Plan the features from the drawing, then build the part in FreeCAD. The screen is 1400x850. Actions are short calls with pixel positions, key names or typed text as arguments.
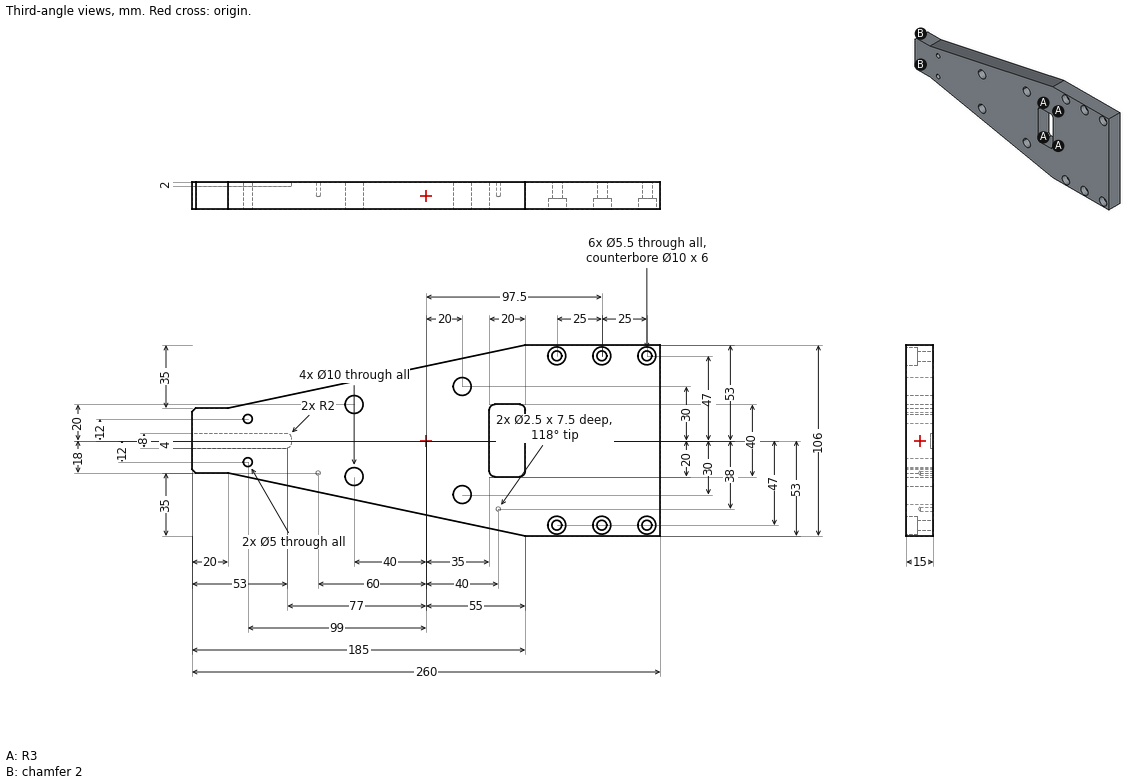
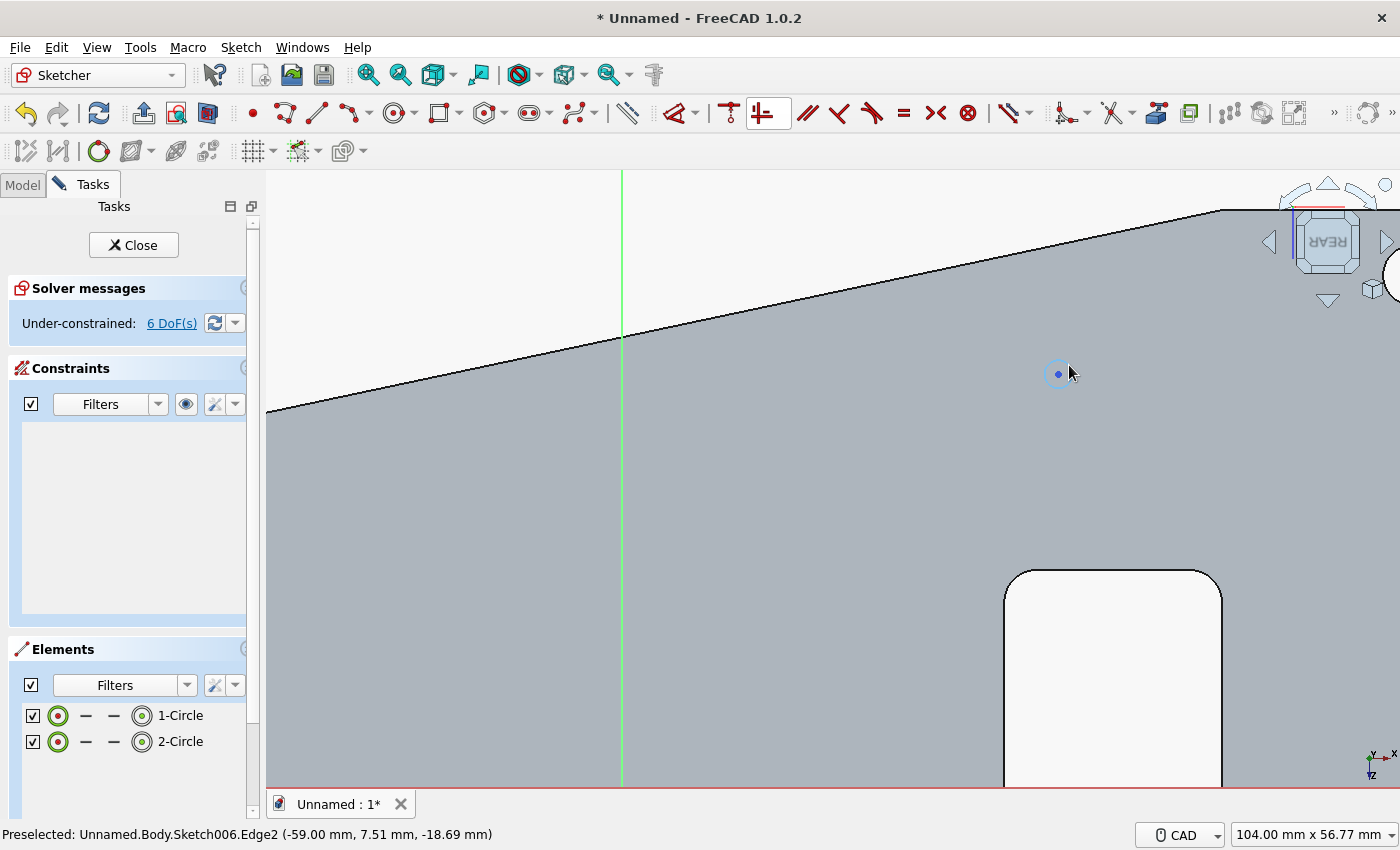
click(1068, 364)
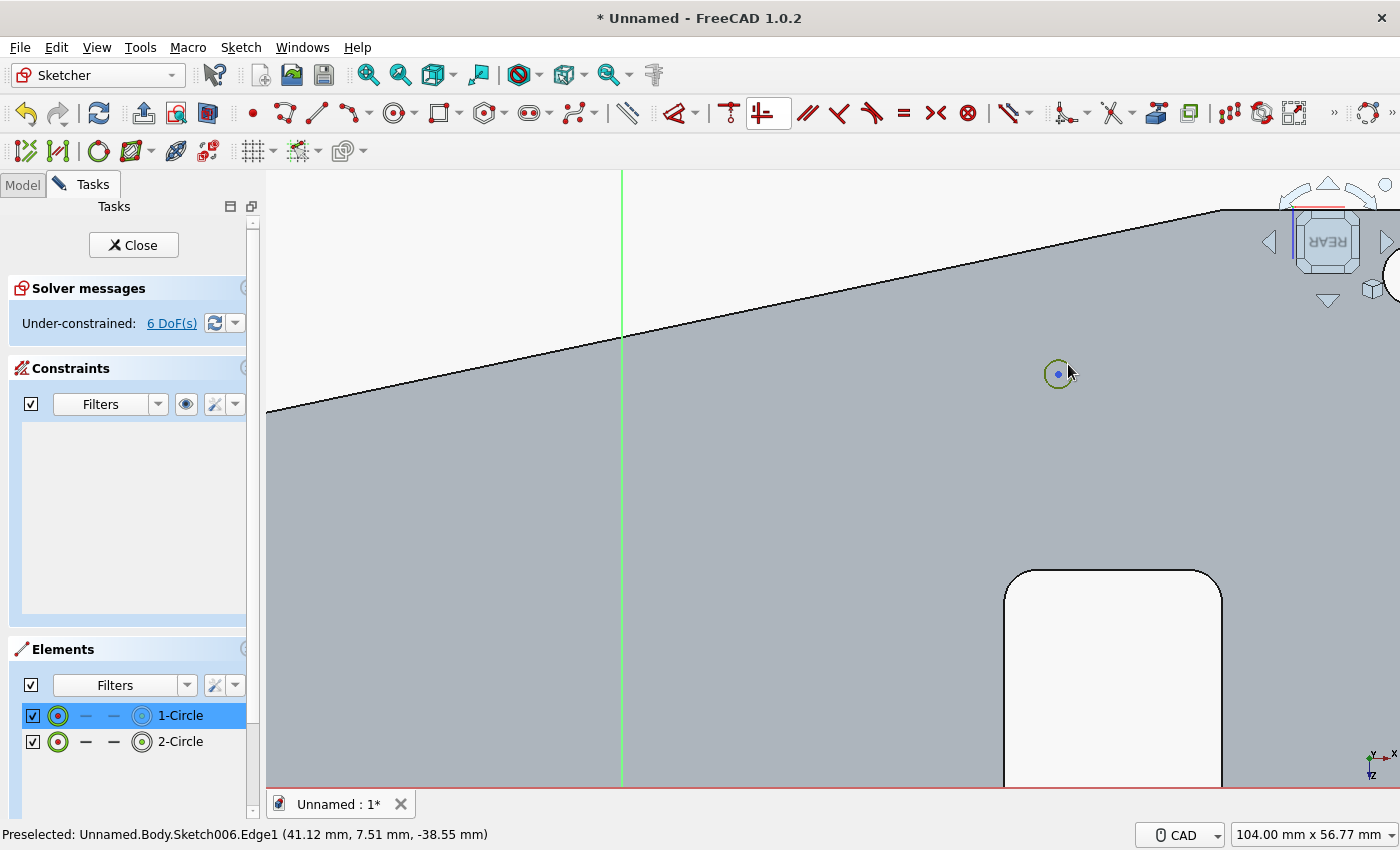
scroll(1070, 365, down, 3)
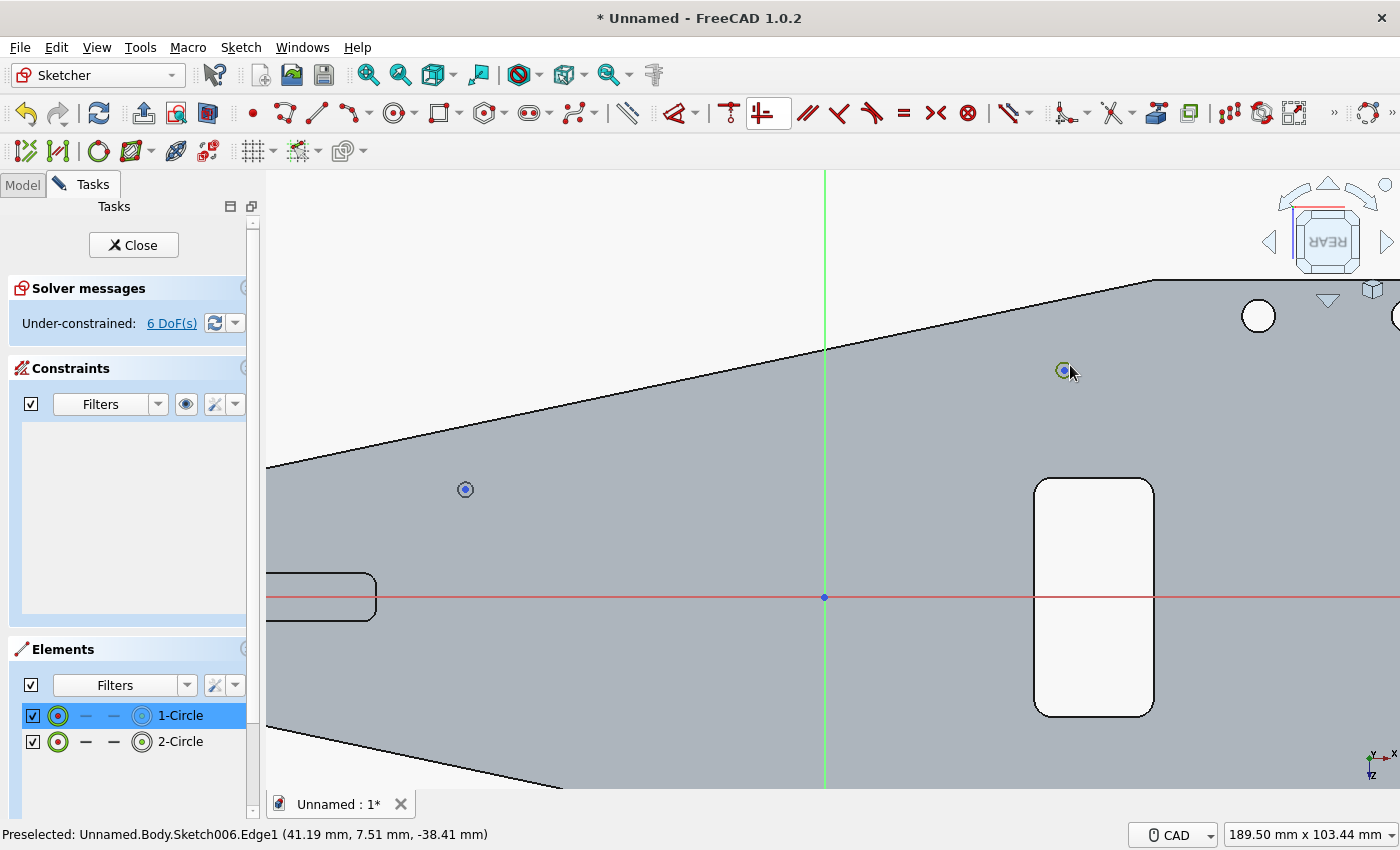
scroll(471, 484, up, 4)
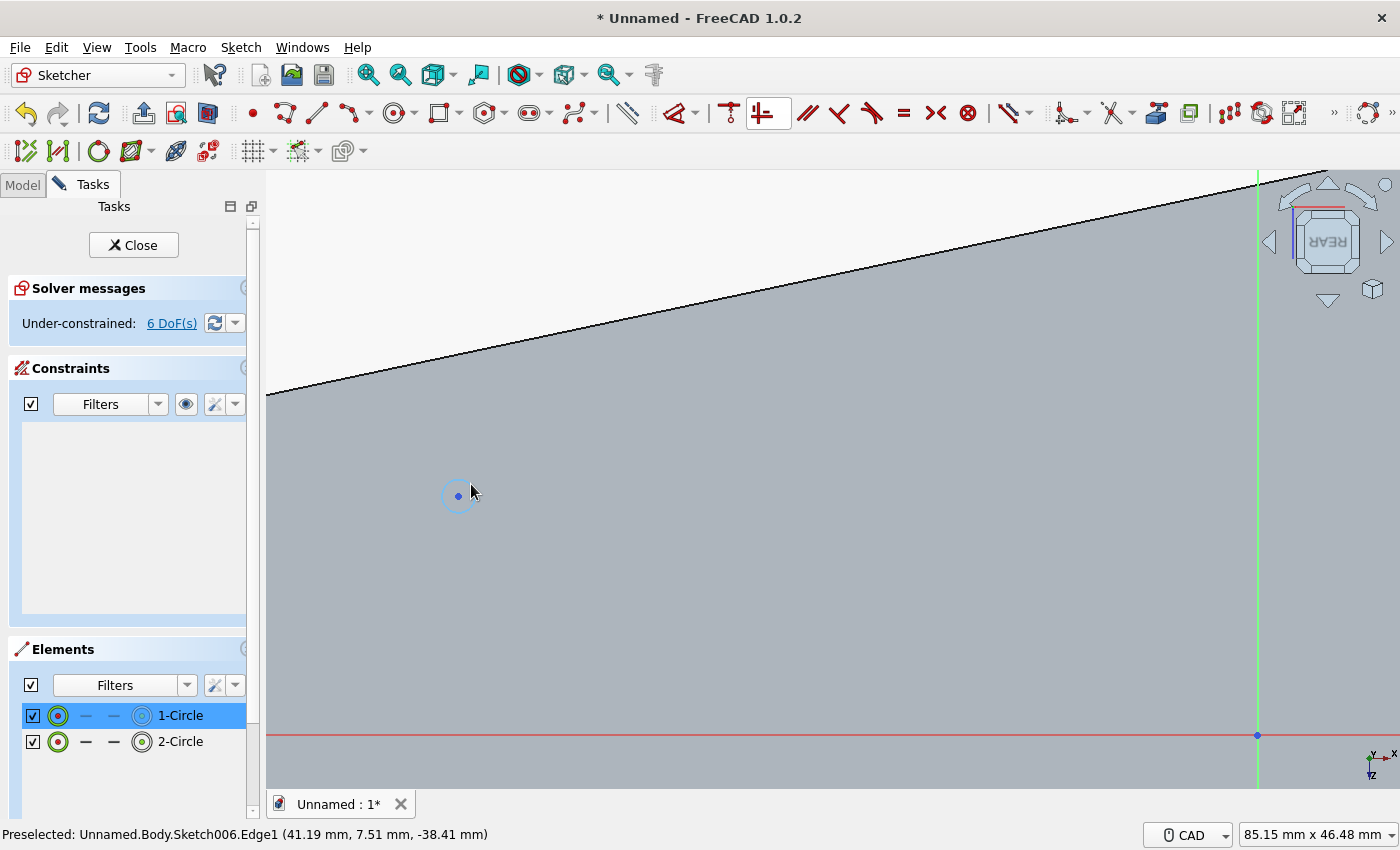
click(470, 484)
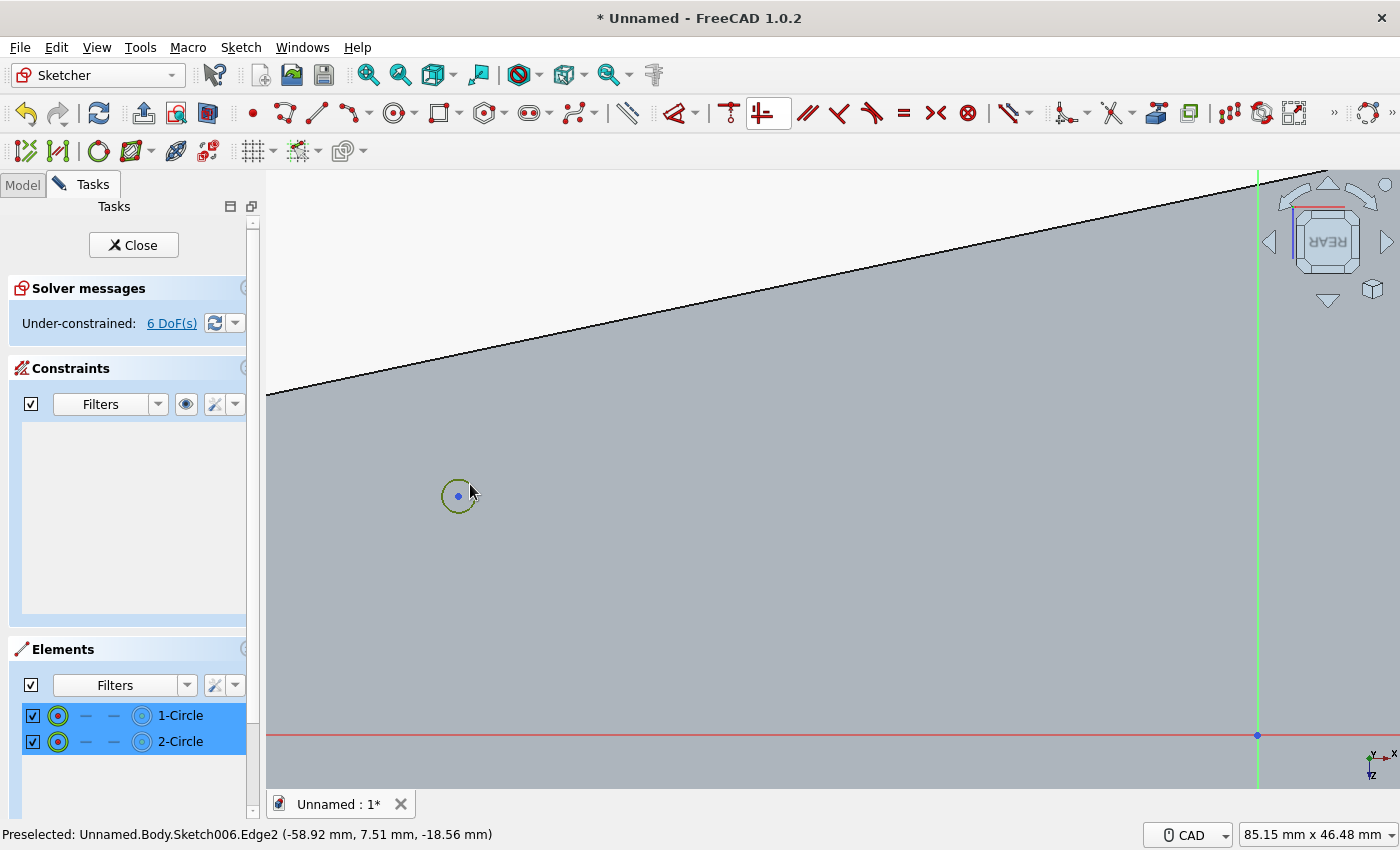
click(904, 114)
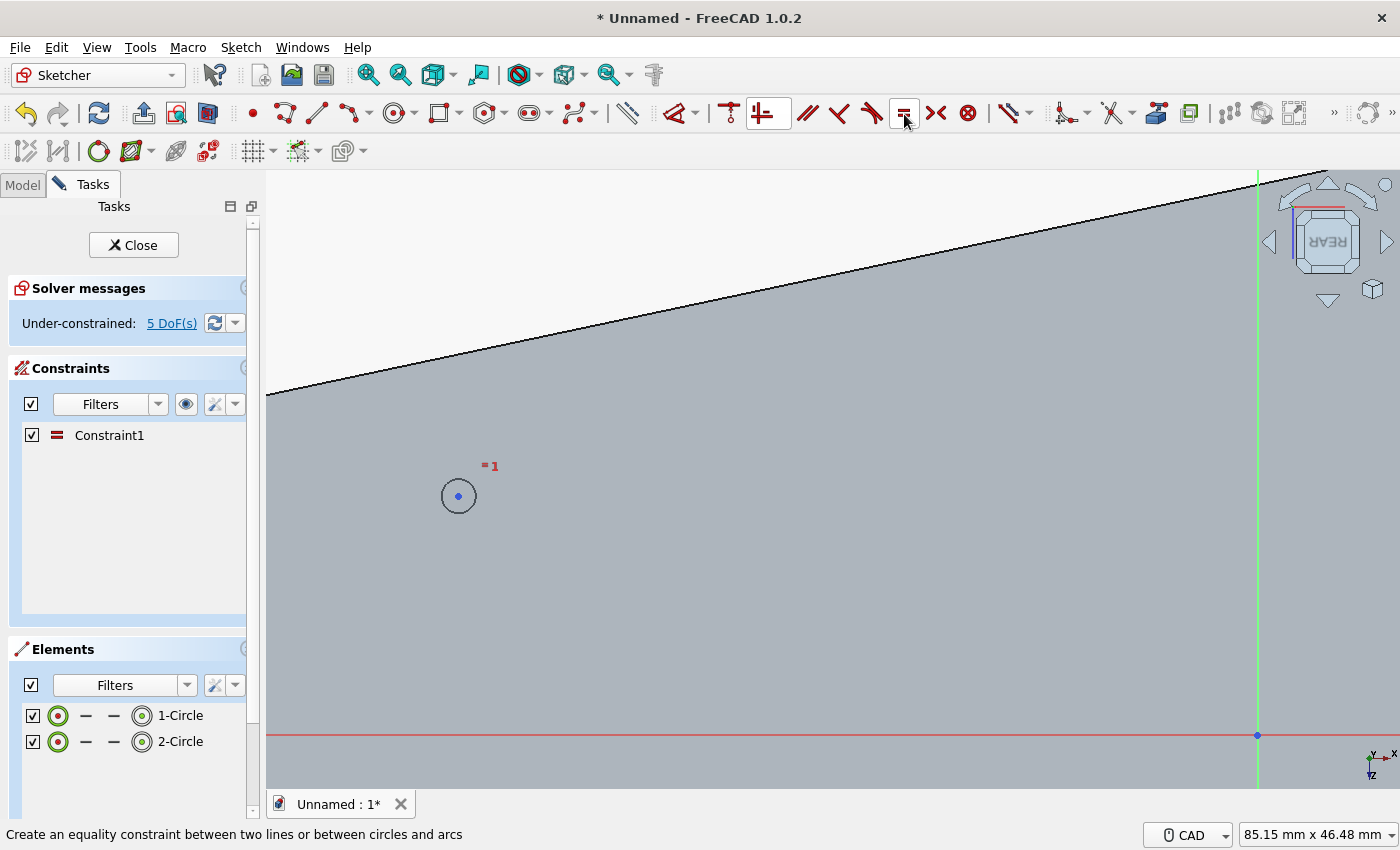
click(674, 114)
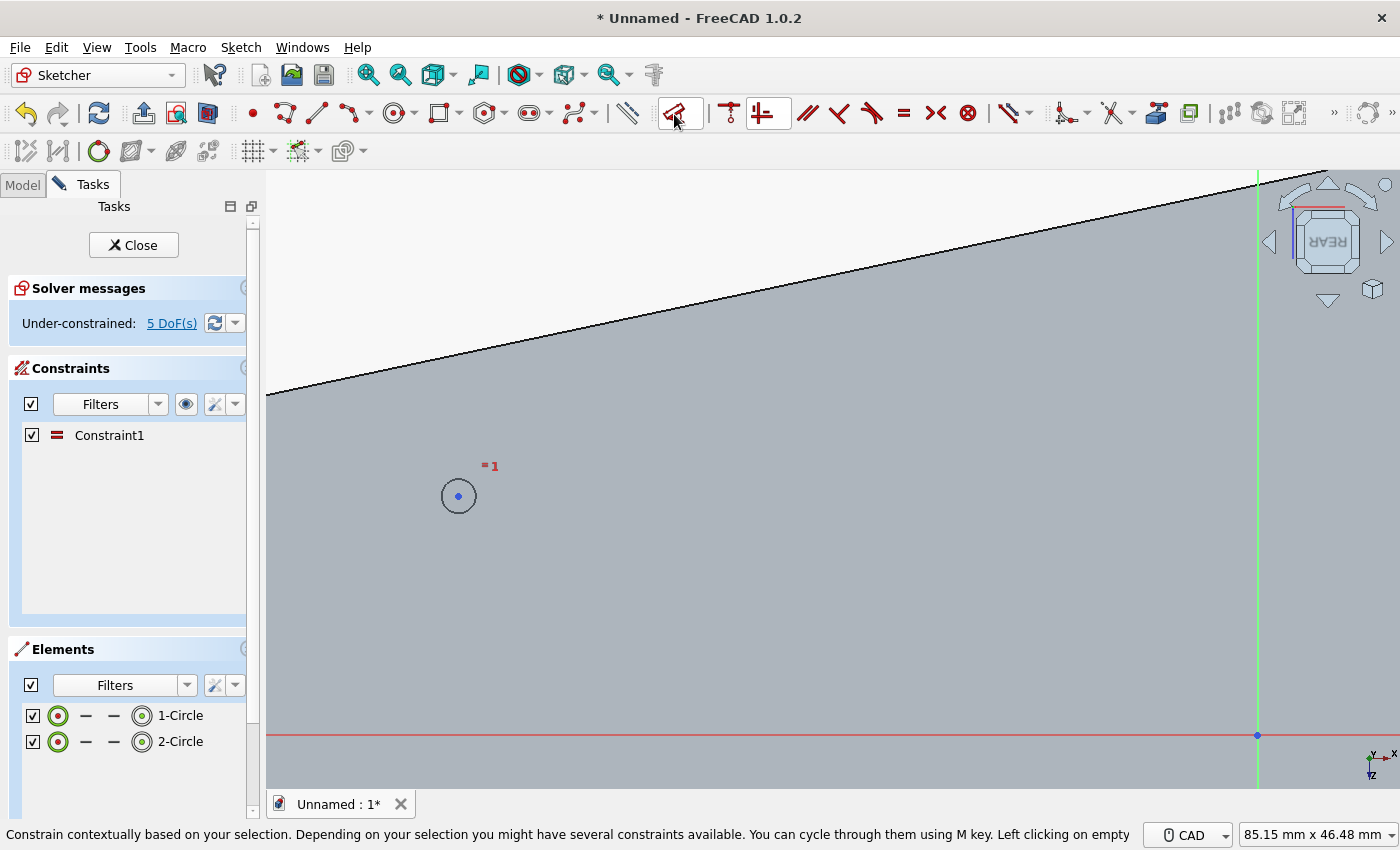
scroll(471, 484, down, 4)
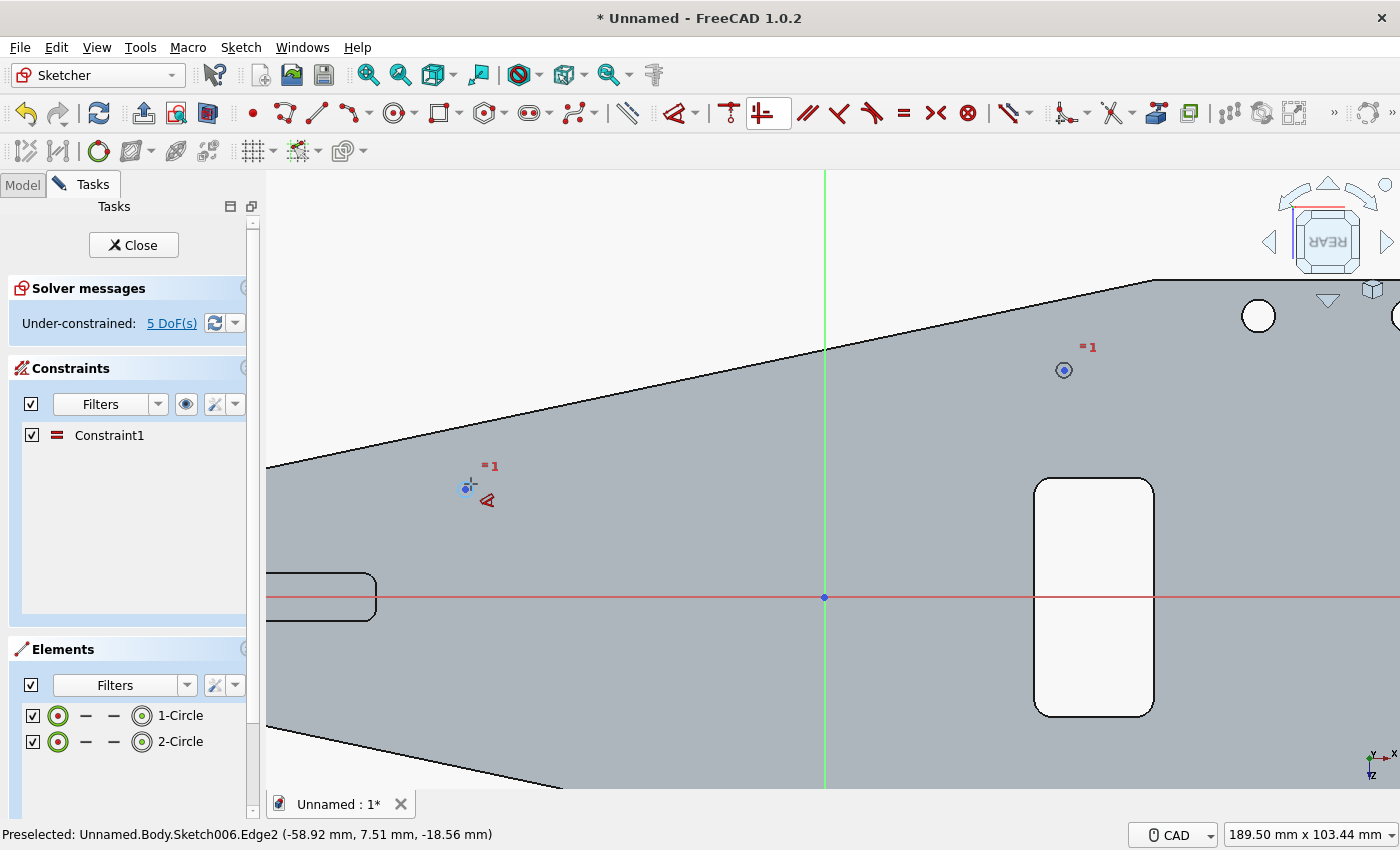
scroll(1069, 365, up, 5)